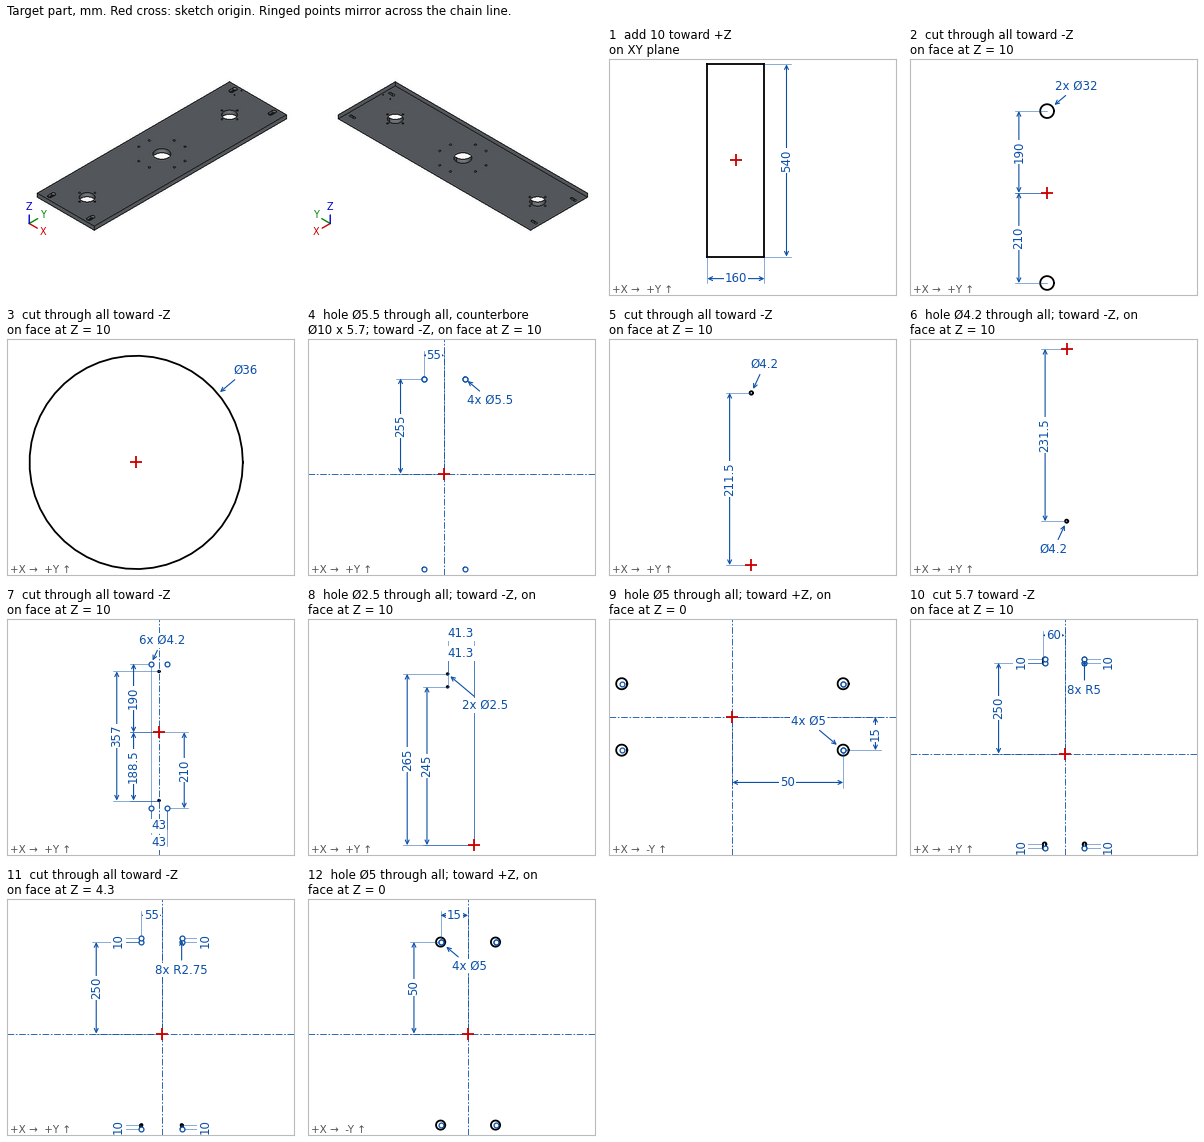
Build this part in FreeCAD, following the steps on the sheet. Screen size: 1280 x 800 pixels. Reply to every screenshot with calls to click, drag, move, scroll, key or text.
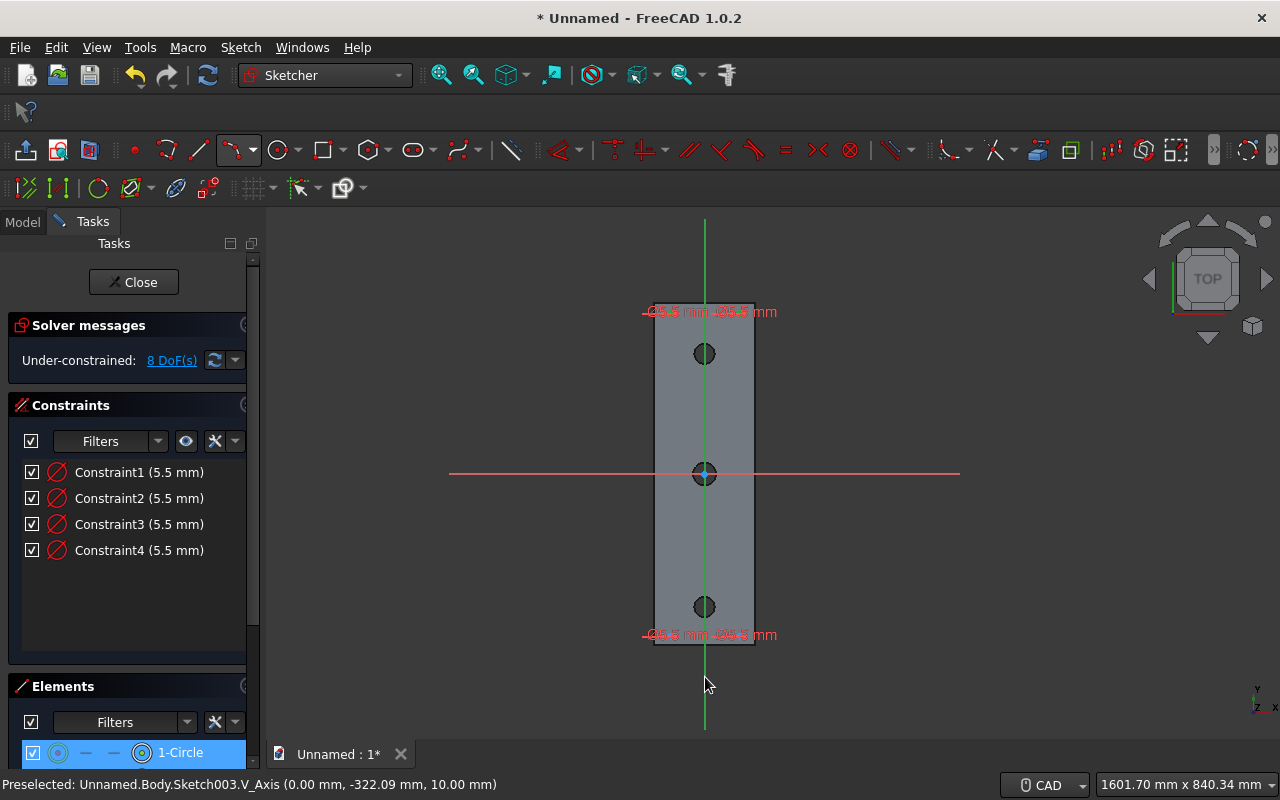
key(s)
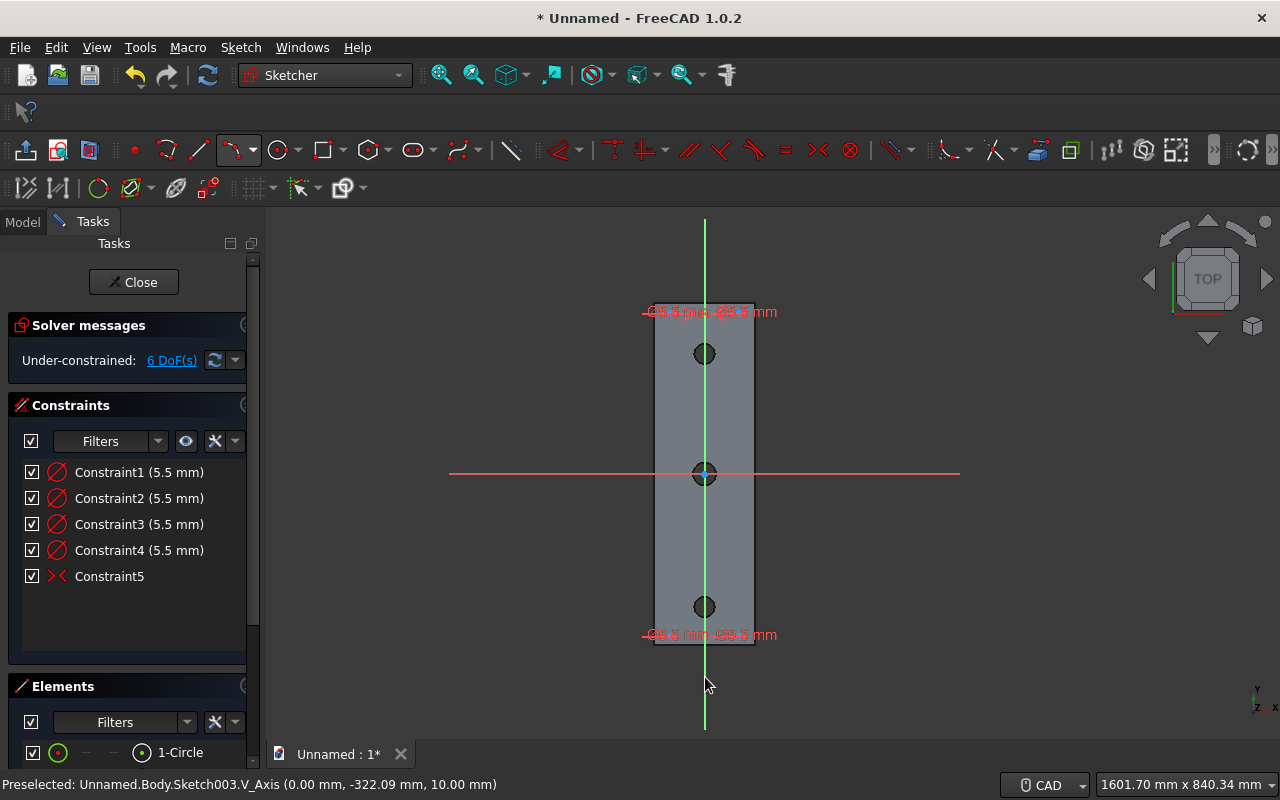
click(739, 314)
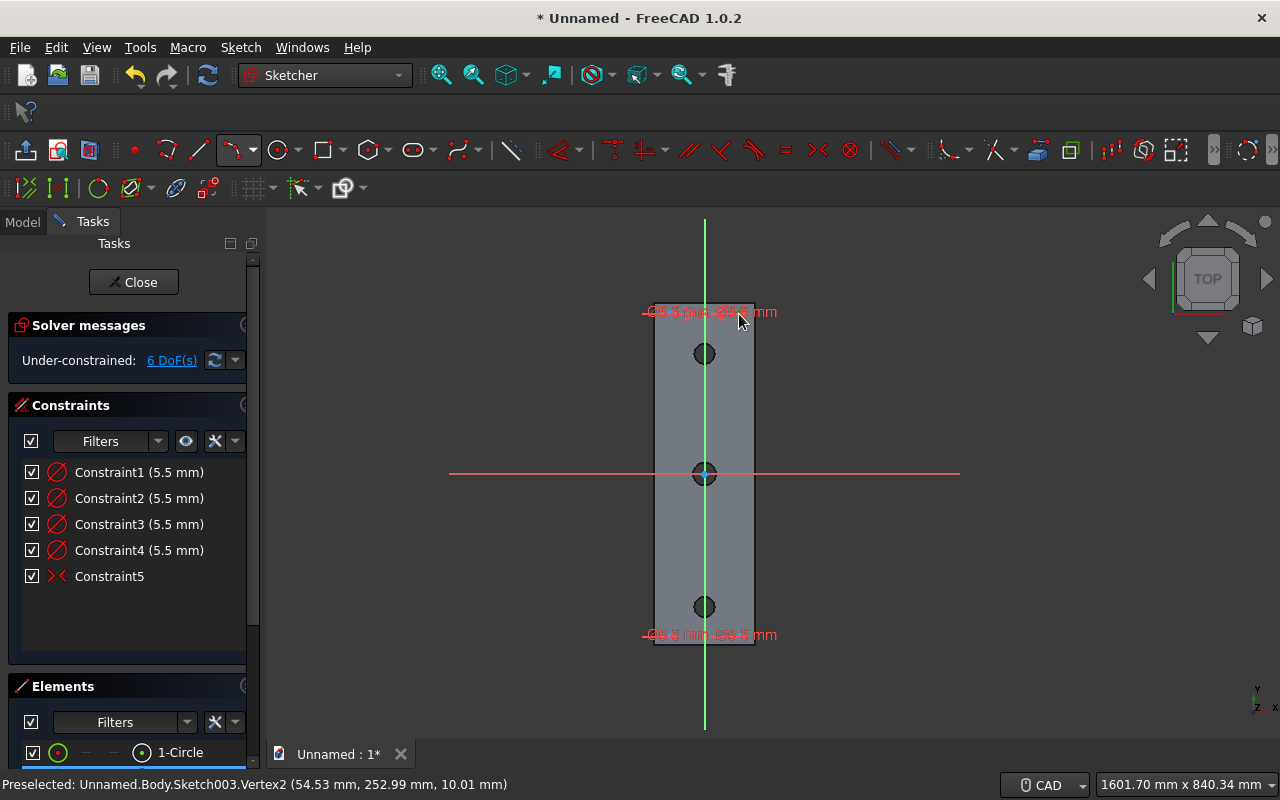
click(739, 637)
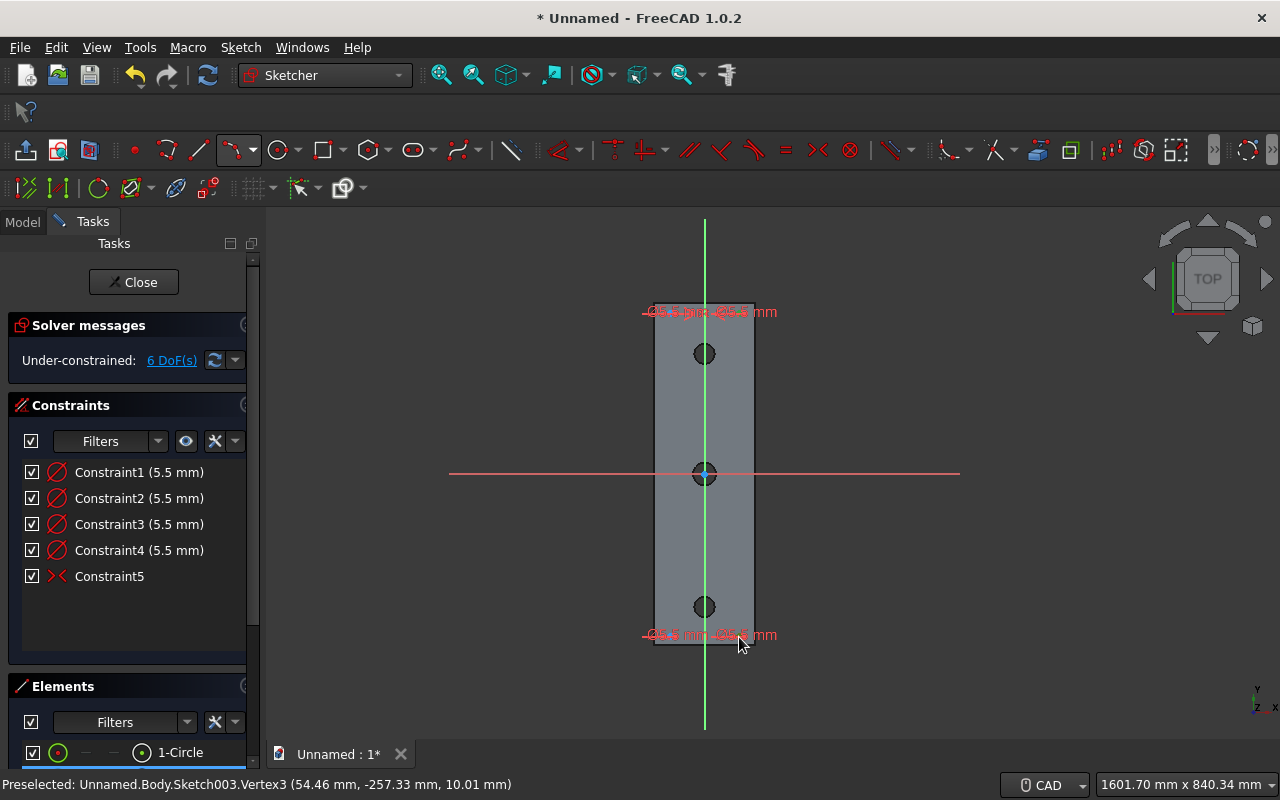
click(470, 474)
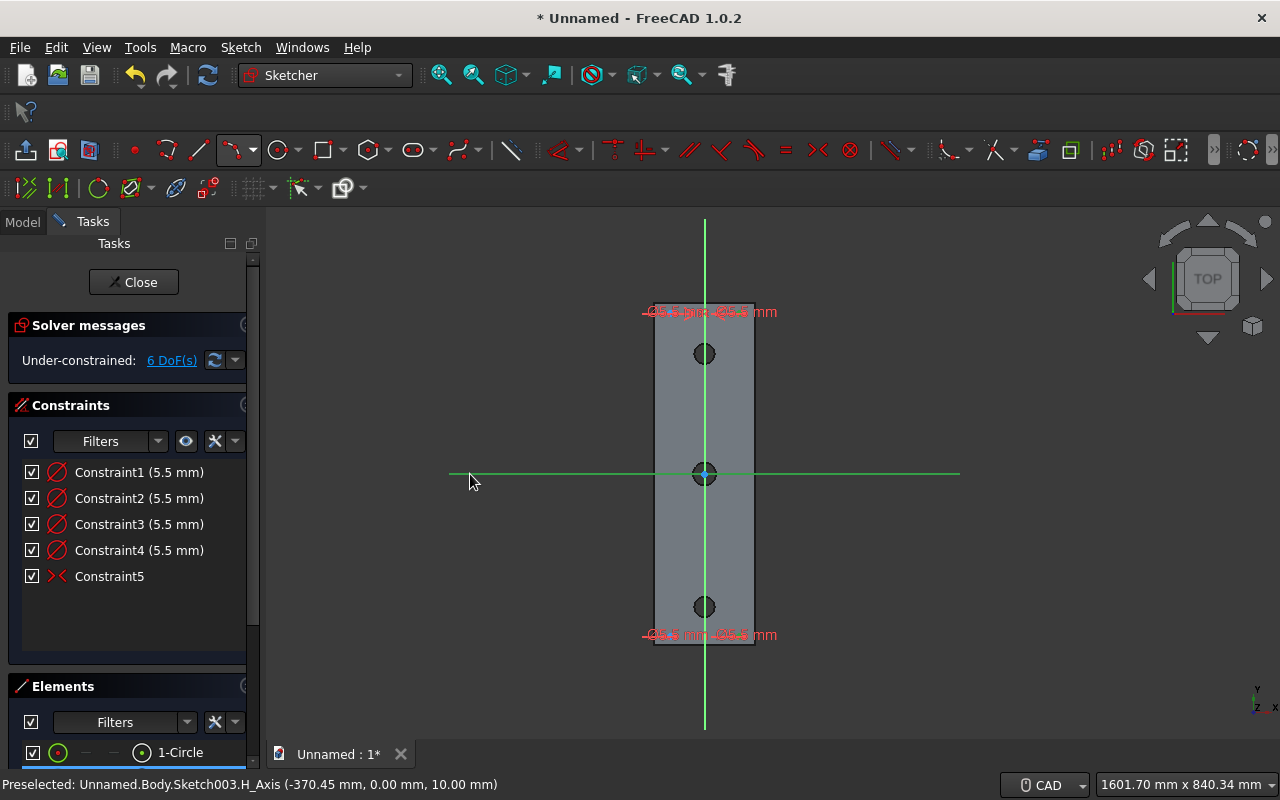
key(s)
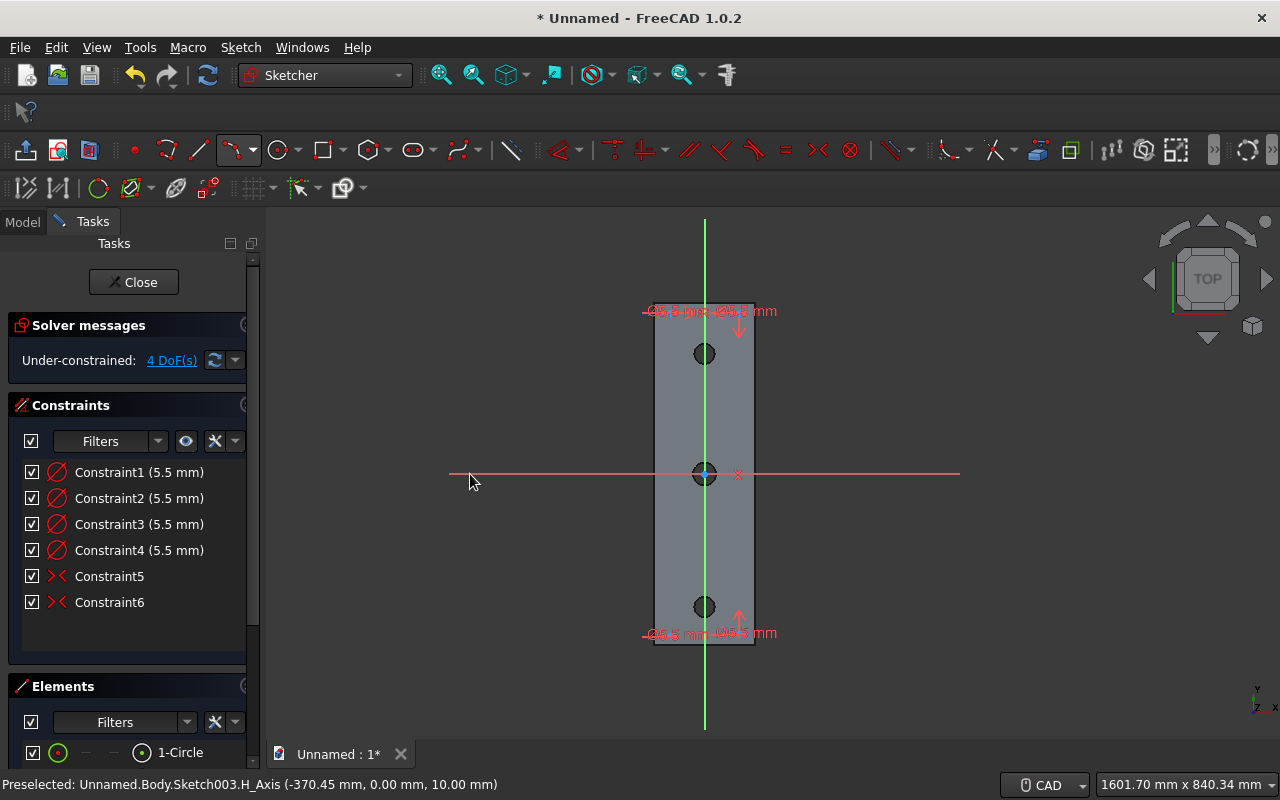
click(670, 313)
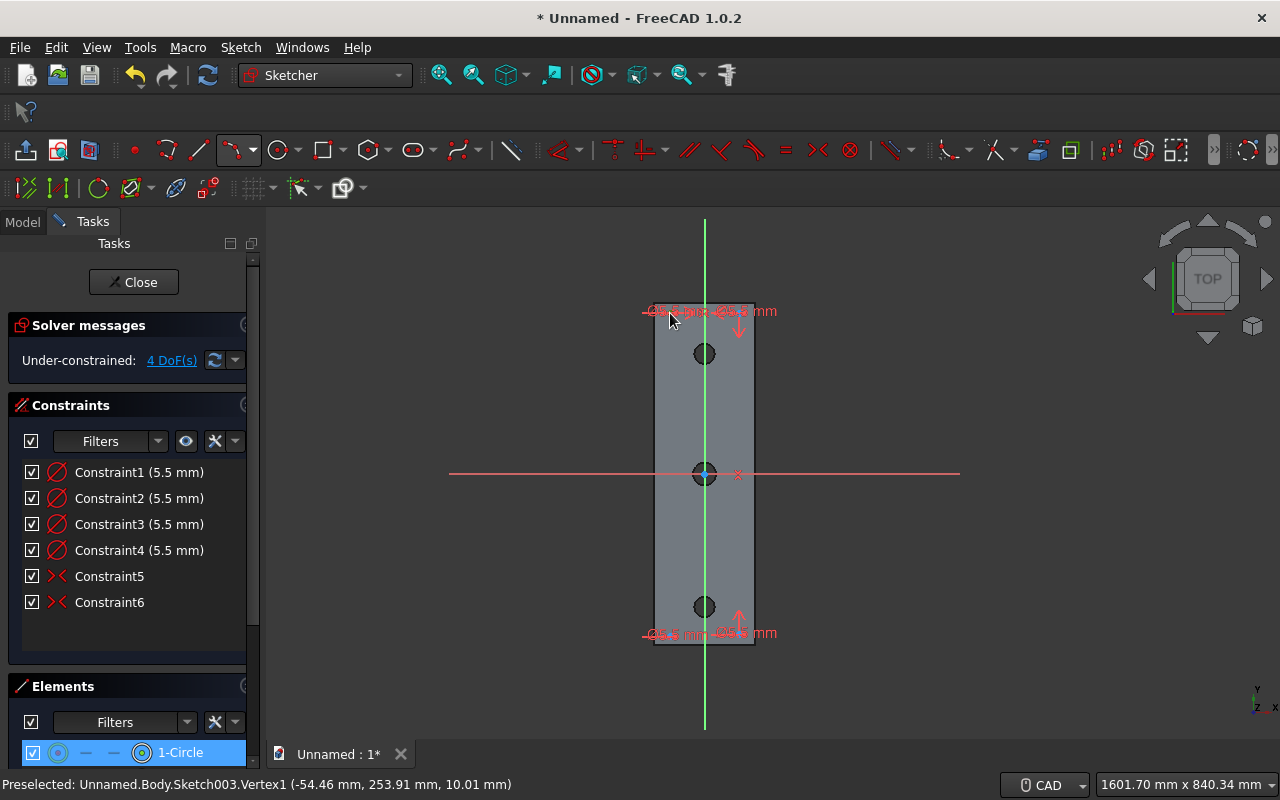
click(670, 637)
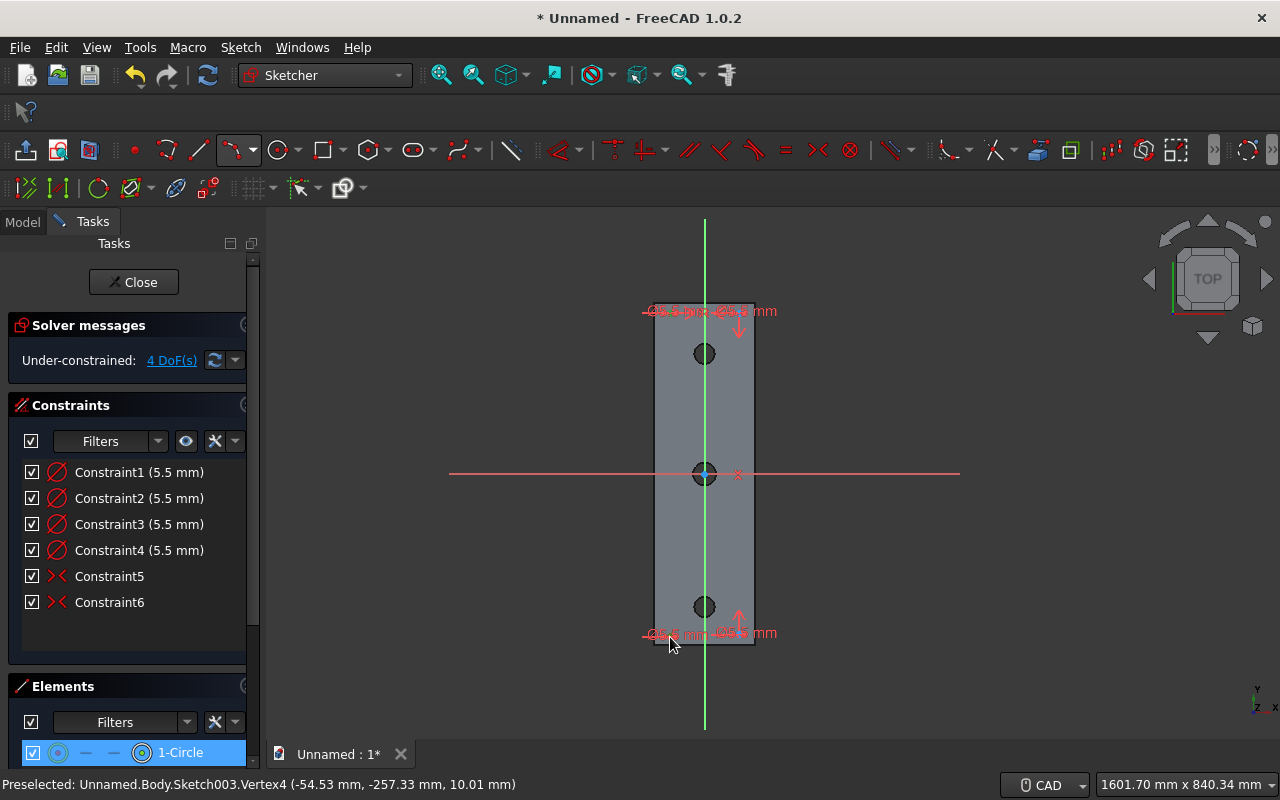
click(470, 474)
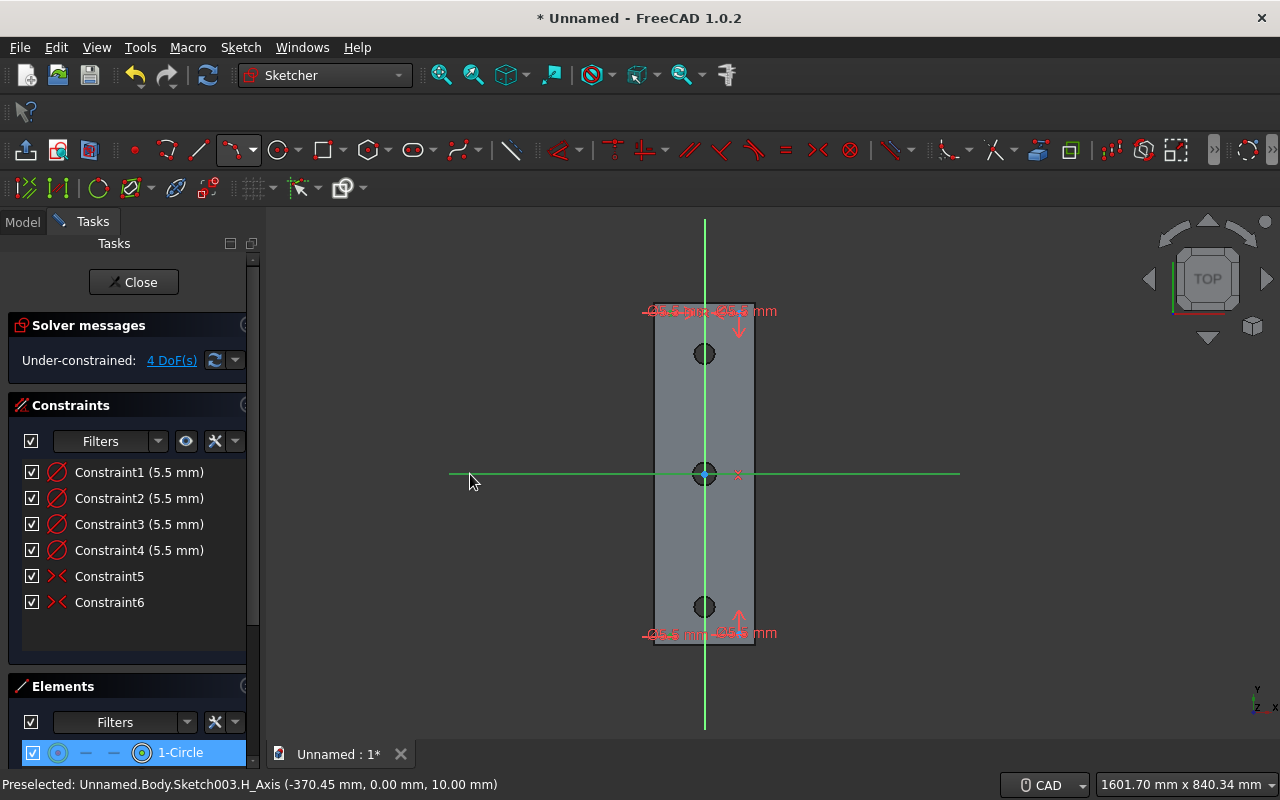
click(818, 150)